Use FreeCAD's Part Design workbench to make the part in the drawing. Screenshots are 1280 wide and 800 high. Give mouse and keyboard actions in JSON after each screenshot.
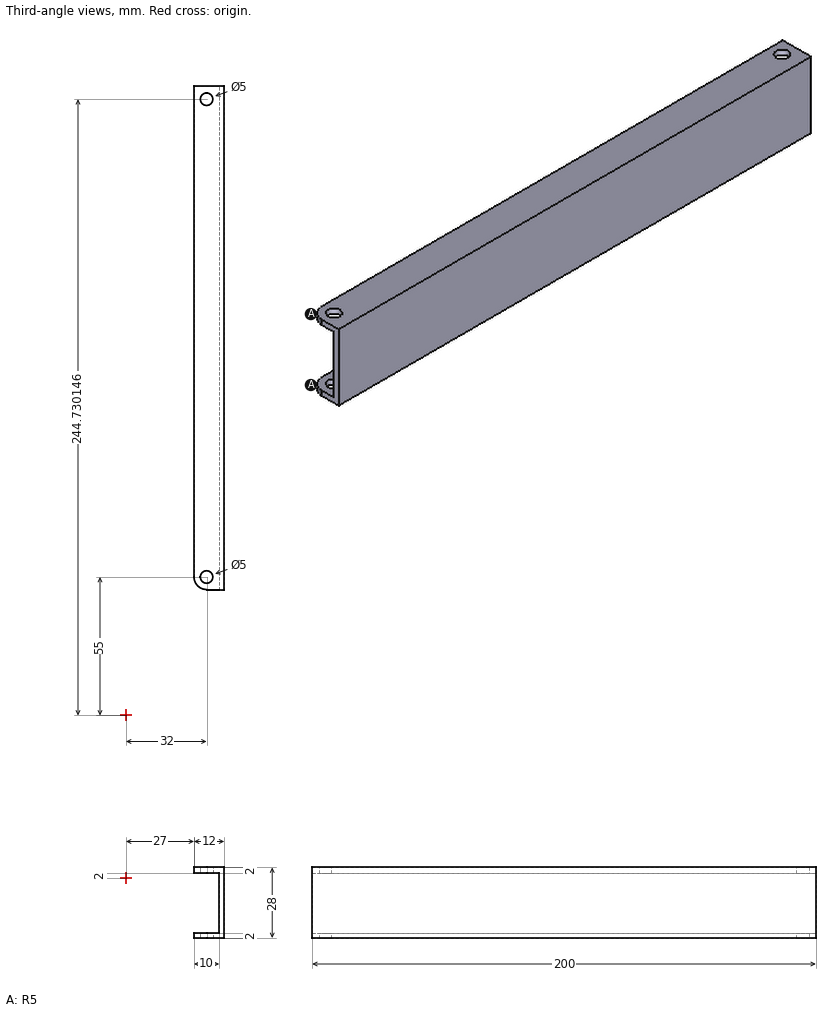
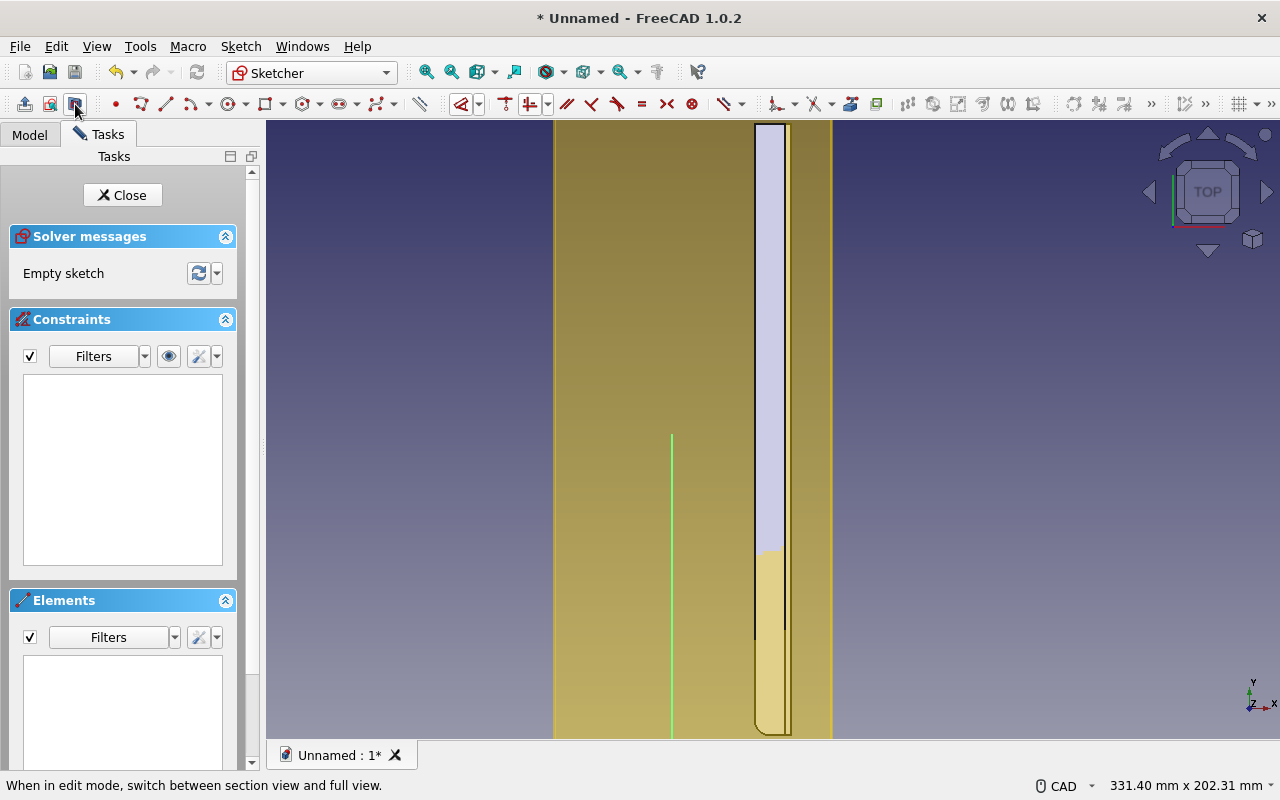
{"action": "scroll", "coordinate": [704, 430], "scroll_direction": "down", "scroll_amount": 5}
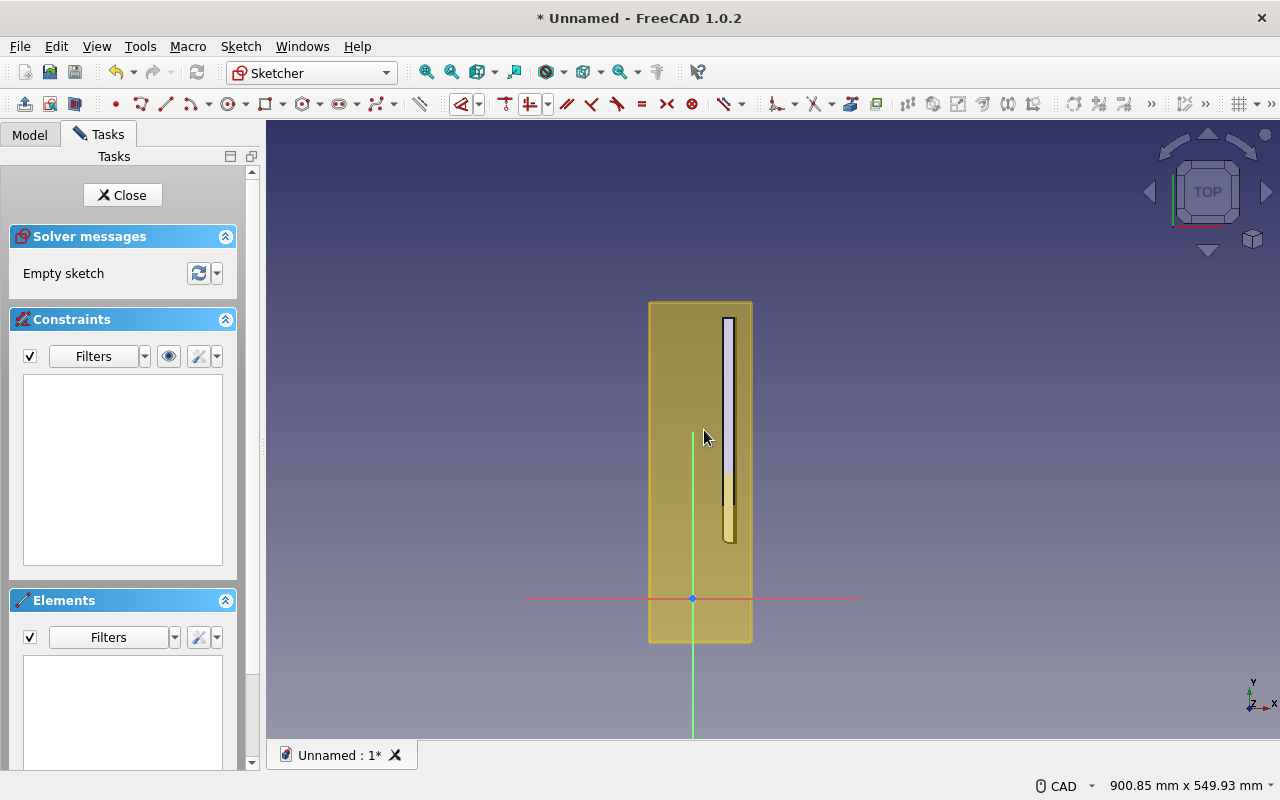
{"action": "scroll", "coordinate": [730, 543], "scroll_direction": "up", "scroll_amount": 15}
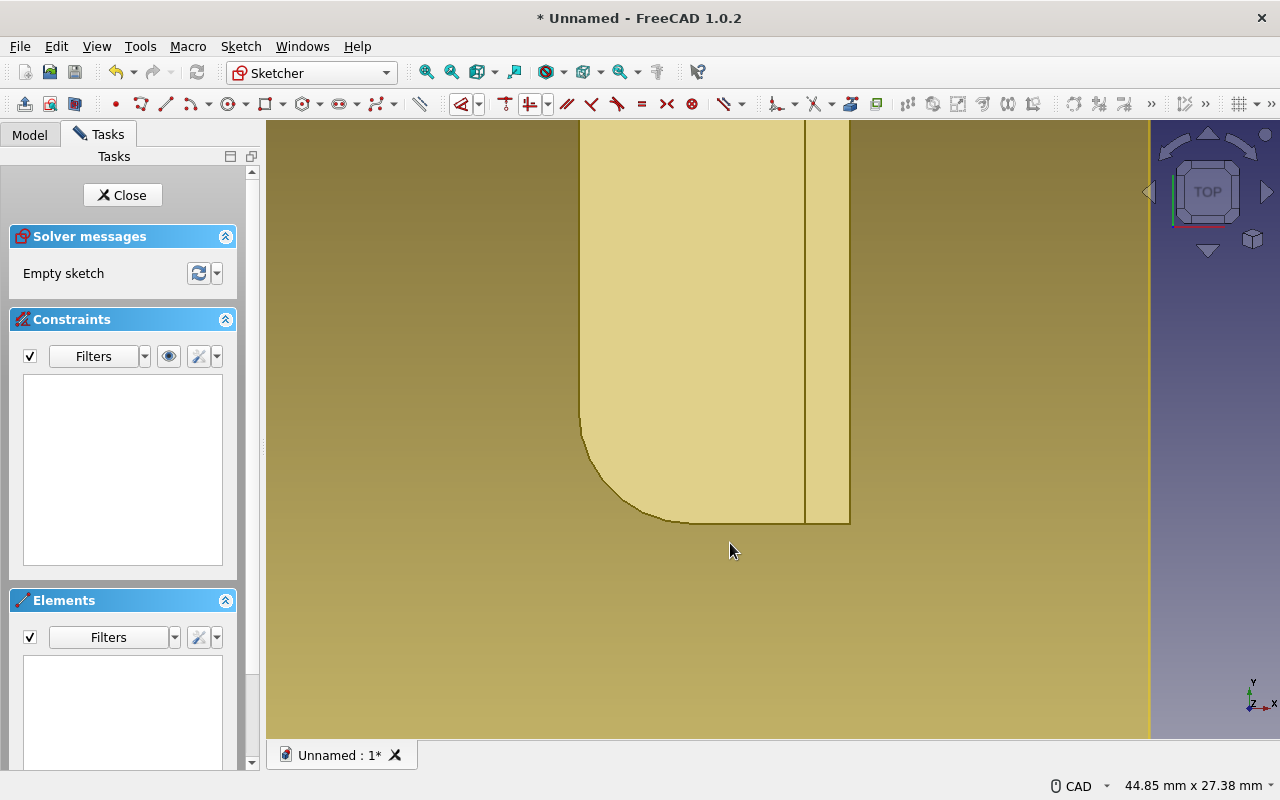
{"action": "scroll", "coordinate": [686, 403], "scroll_direction": "up", "scroll_amount": 6}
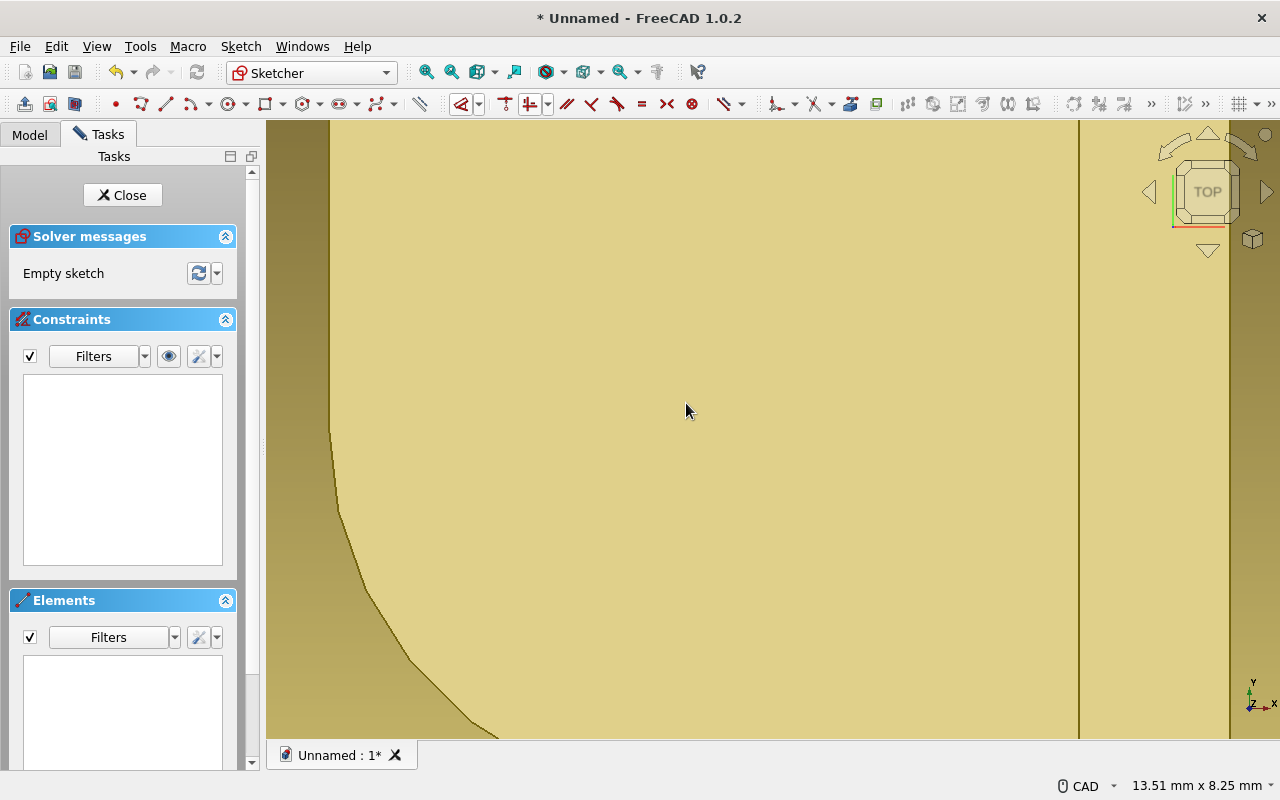
{"action": "left_click", "coordinate": [228, 104]}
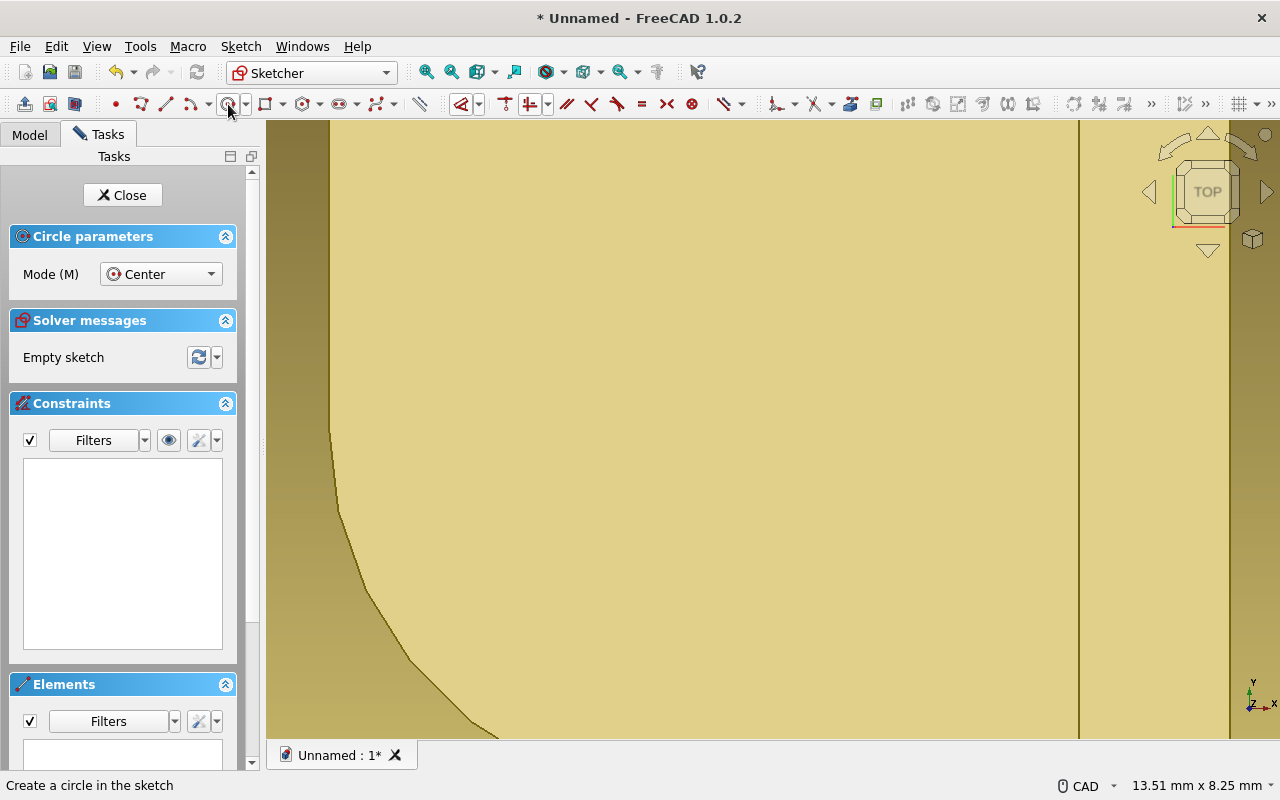
{"action": "left_click", "coordinate": [704, 428]}
{"action": "left_click", "coordinate": [837, 295]}
{"action": "key", "text": "Escape"}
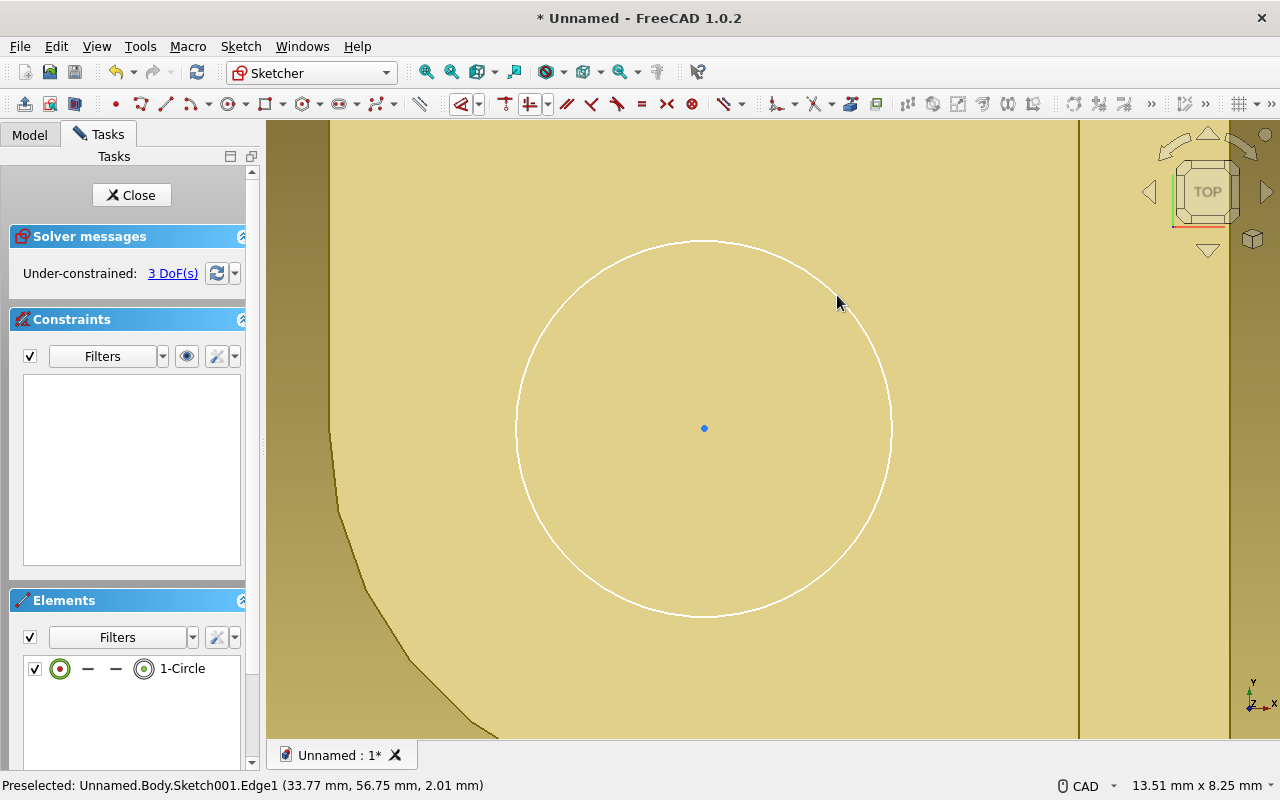
{"action": "left_click", "coordinate": [837, 296]}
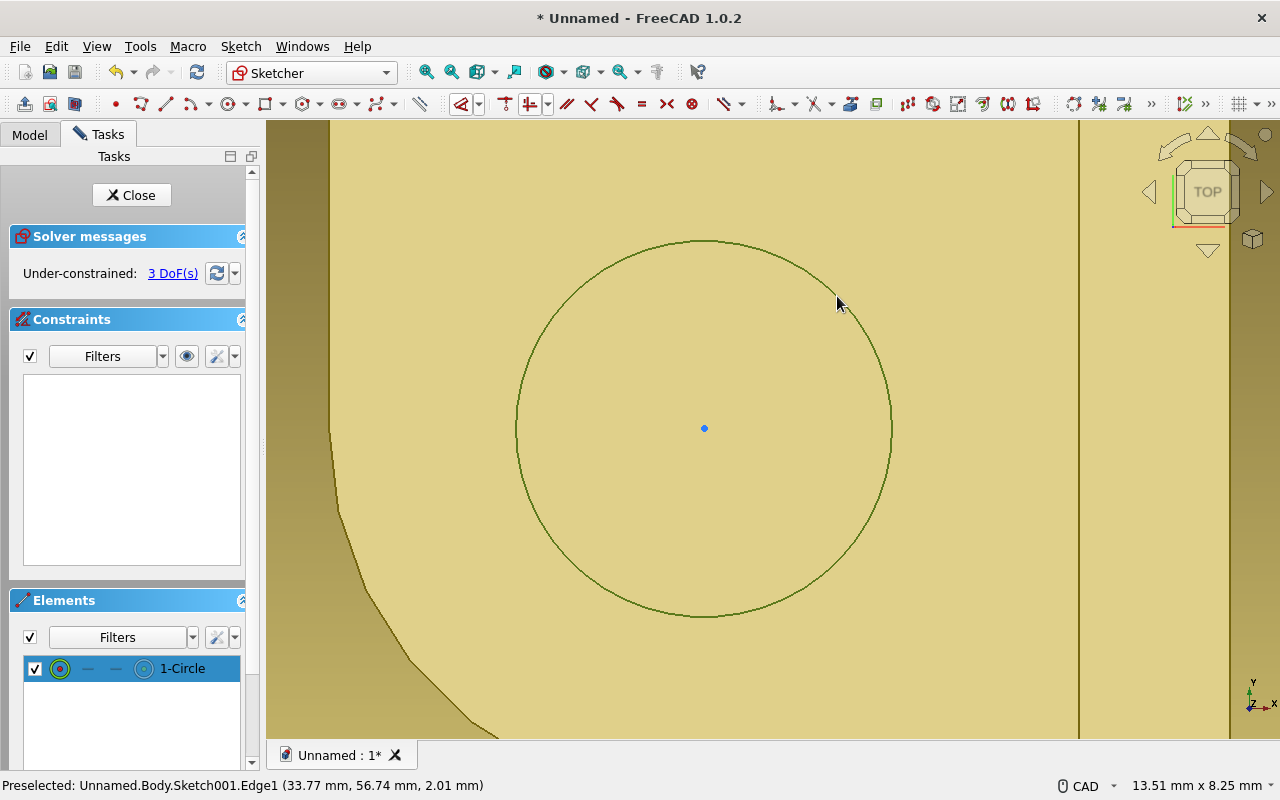
{"action": "key", "text": "k o"}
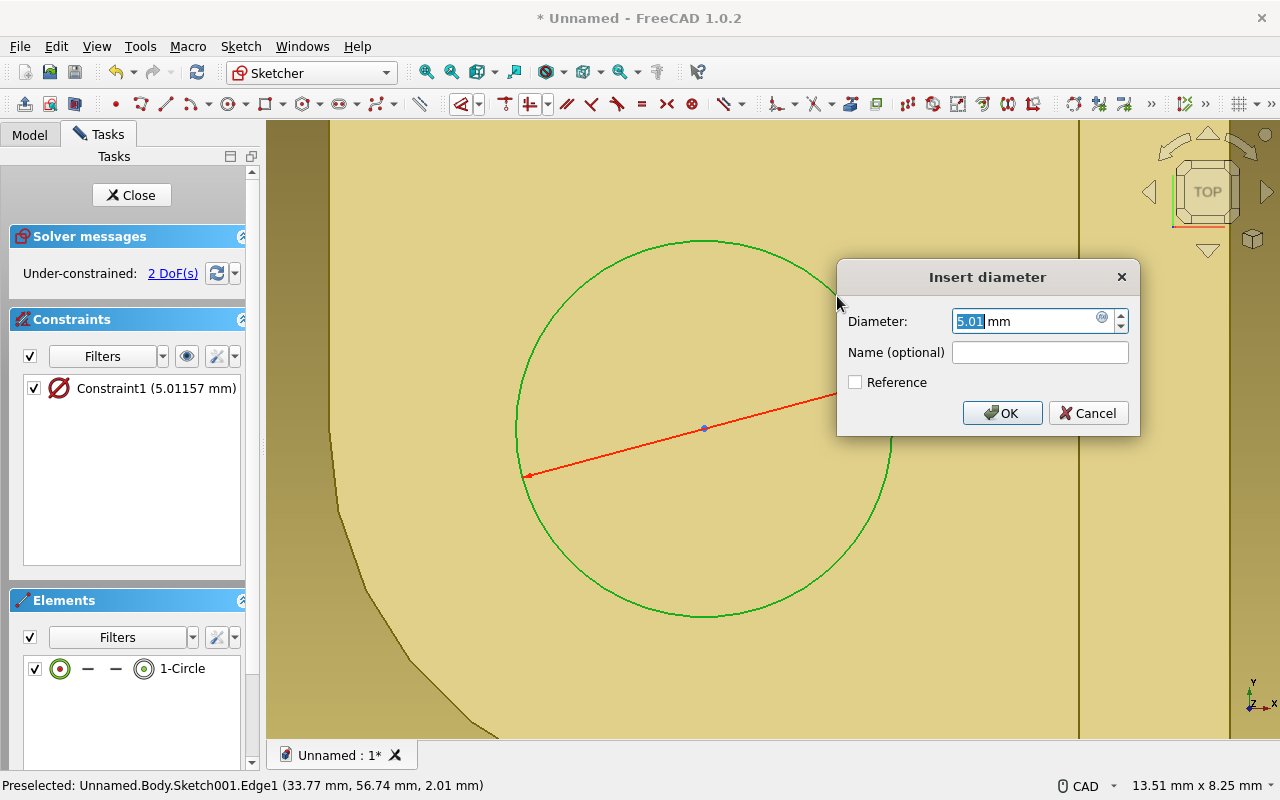
{"action": "type", "text": "5"}
{"action": "key", "text": "Return"}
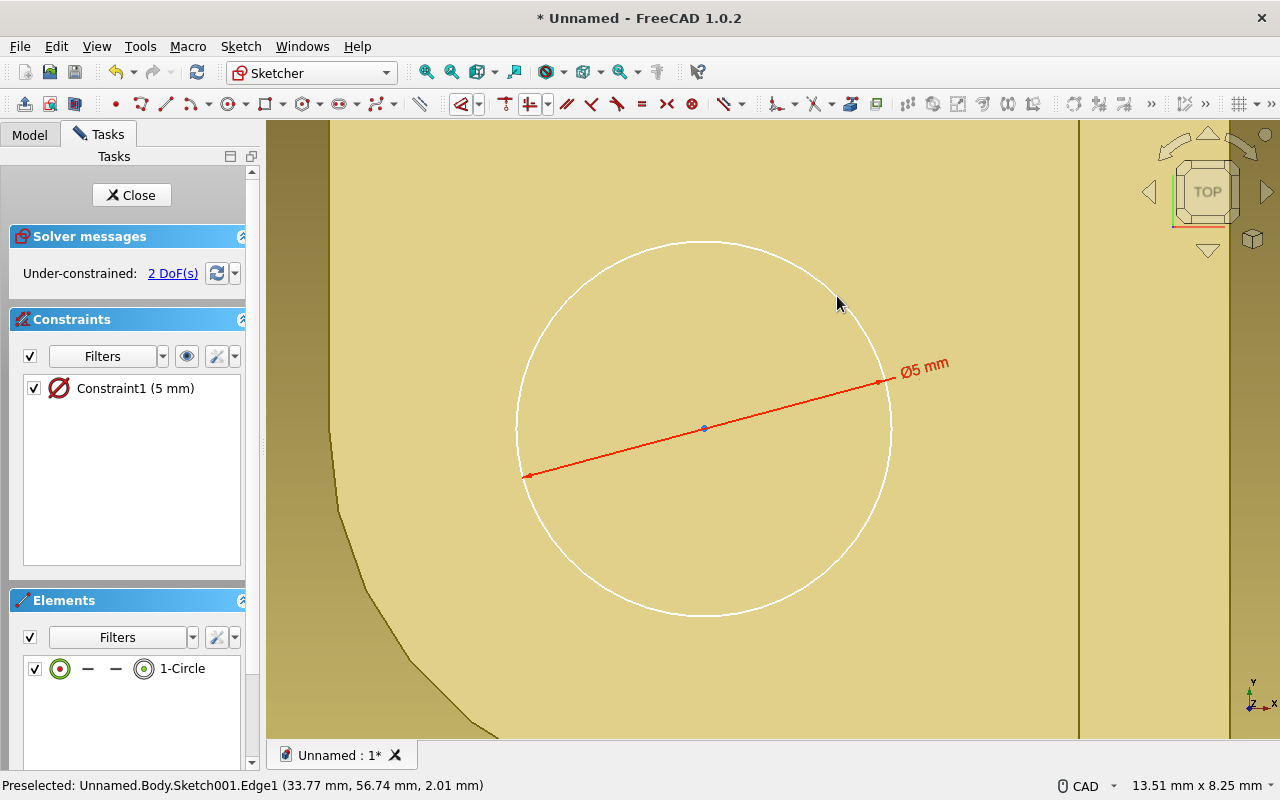
{"action": "left_click", "coordinate": [704, 429]}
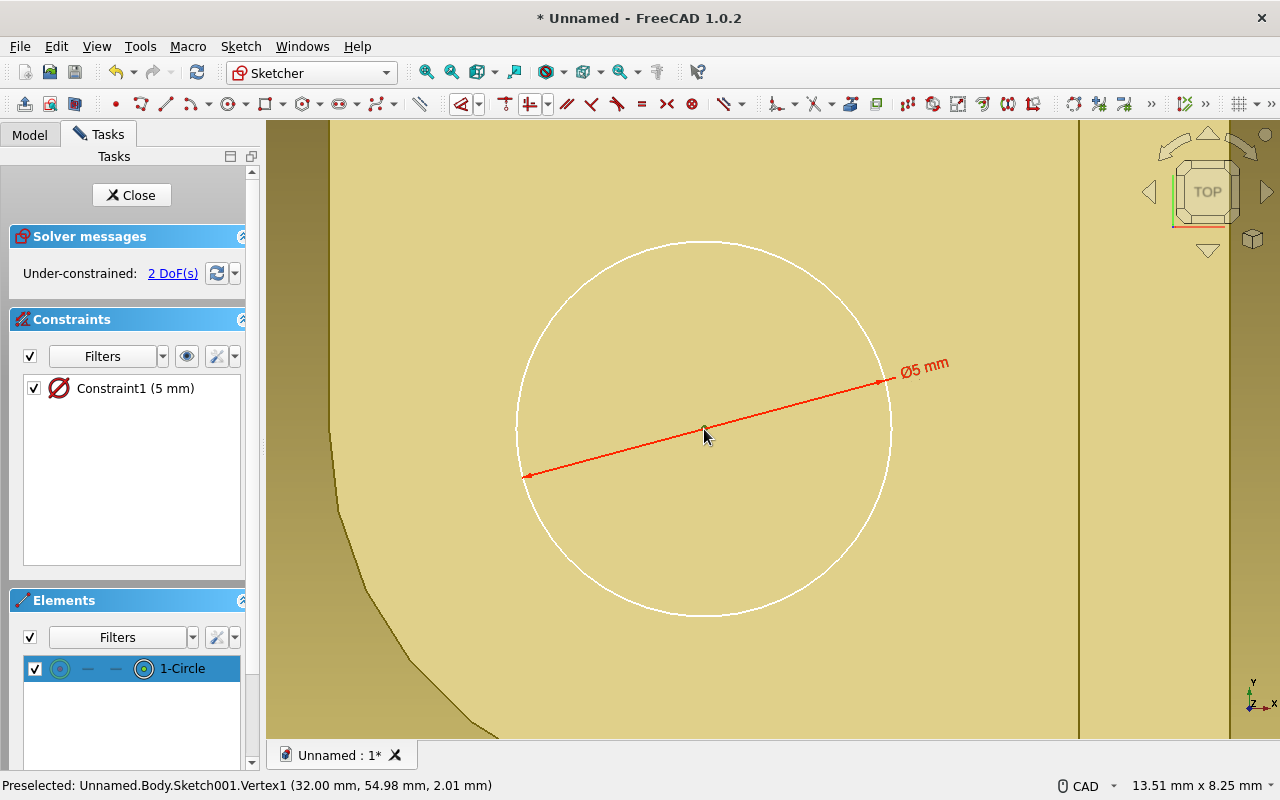
{"action": "left_click", "coordinate": [478, 104]}